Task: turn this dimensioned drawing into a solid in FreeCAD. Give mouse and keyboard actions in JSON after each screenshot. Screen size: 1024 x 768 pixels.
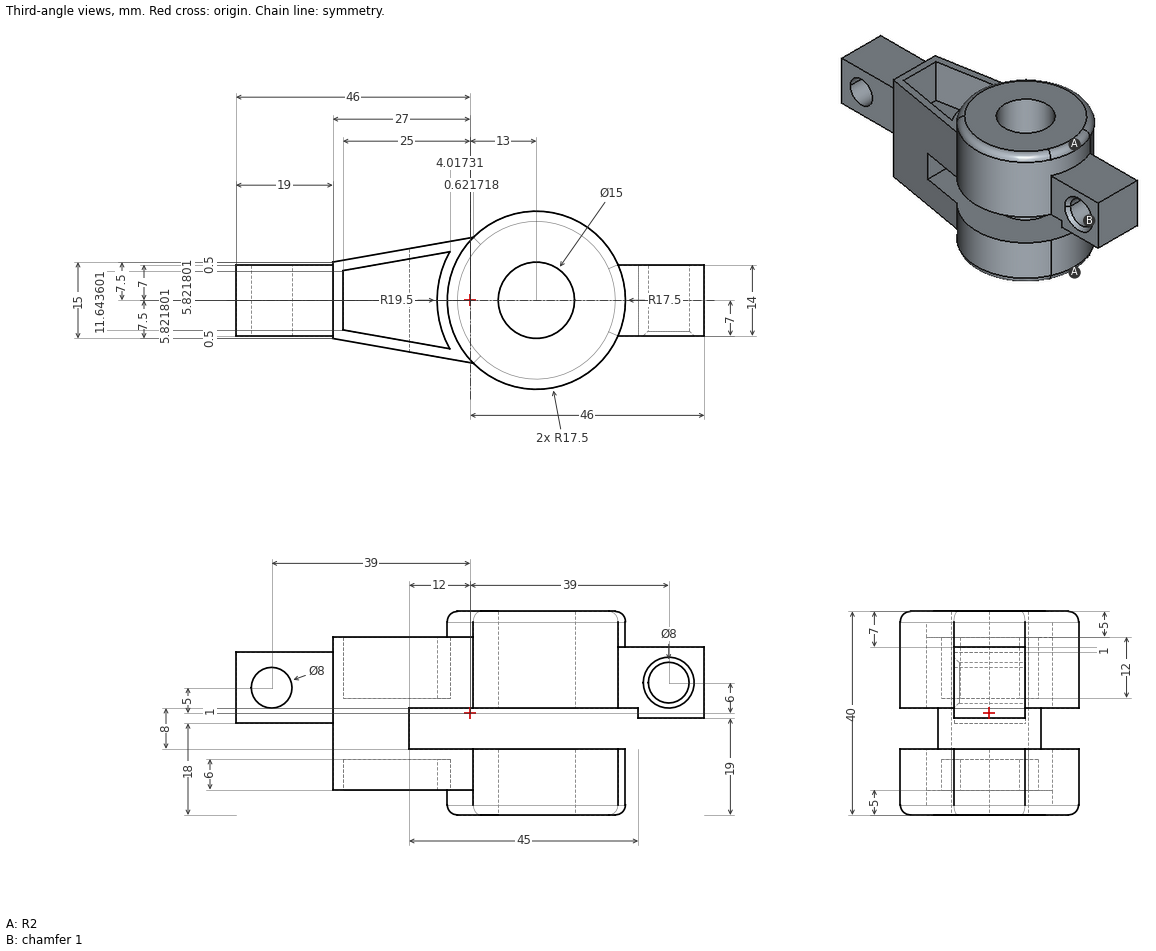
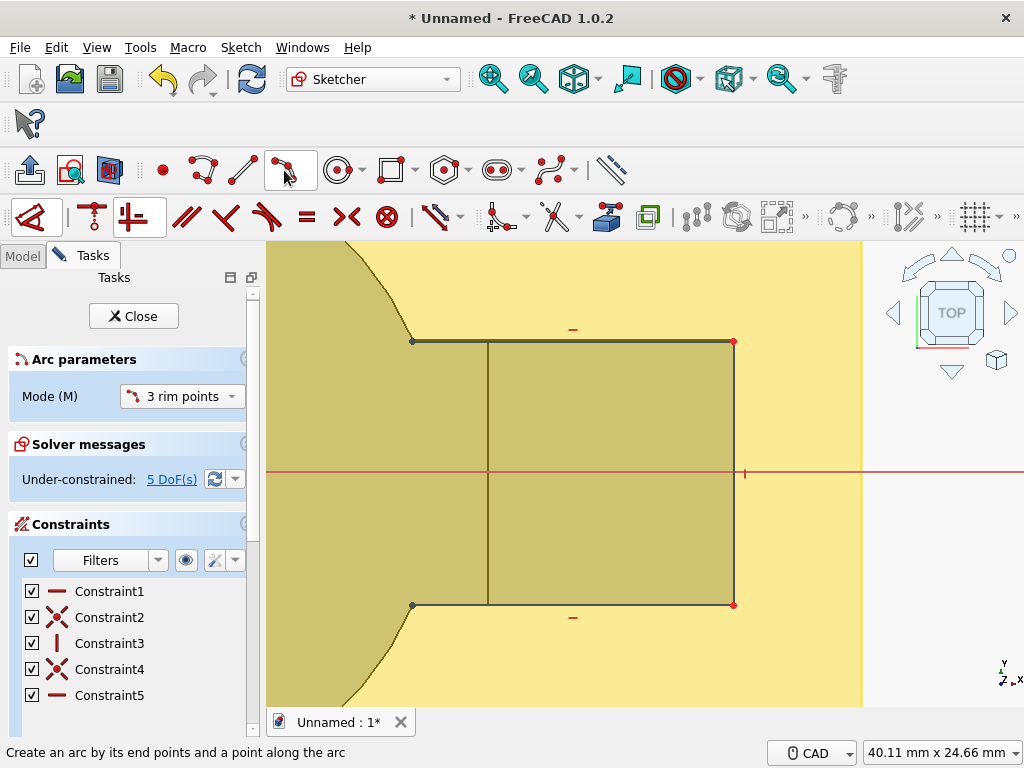
{"action": "left_click", "coordinate": [413, 605]}
{"action": "left_click", "coordinate": [413, 342]}
{"action": "left_click", "coordinate": [440, 500]}
{"action": "key", "text": "Escape"}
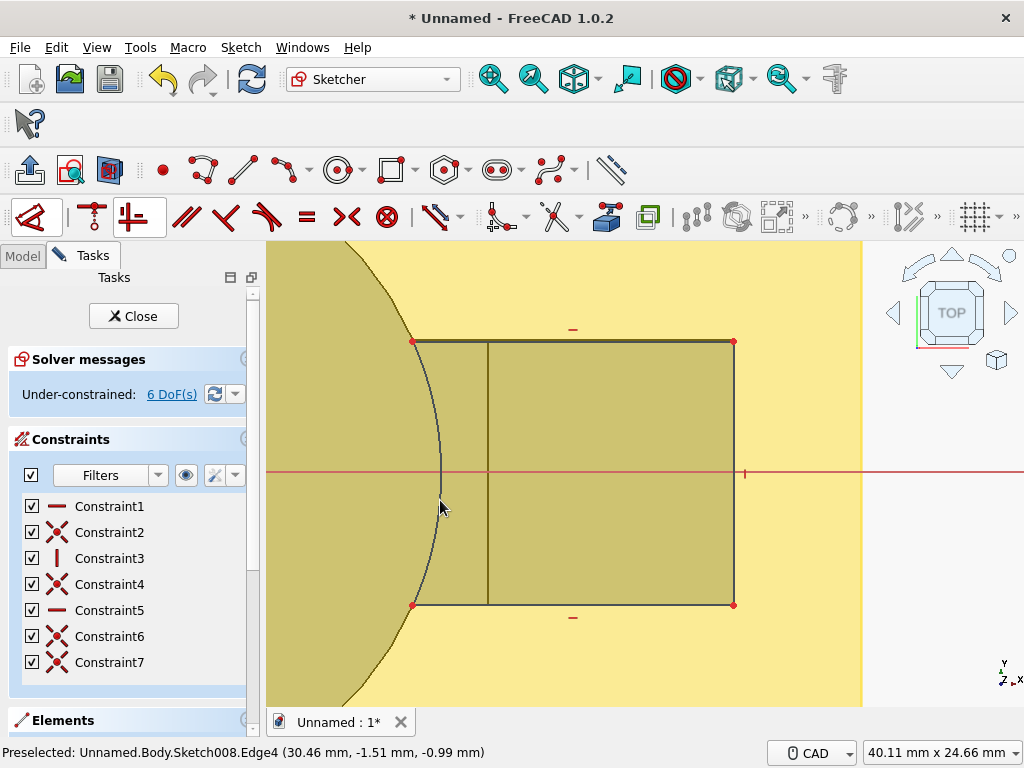
{"action": "scroll", "coordinate": [859, 477], "scroll_direction": "down", "scroll_amount": 2}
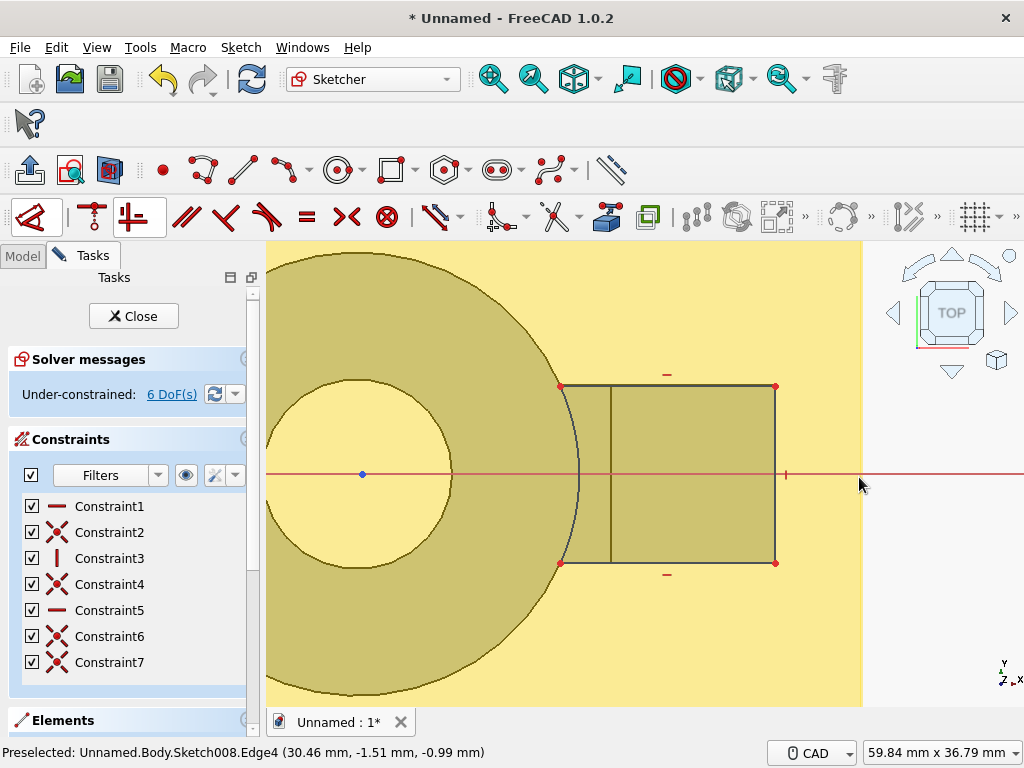
{"action": "left_click", "coordinate": [363, 475]}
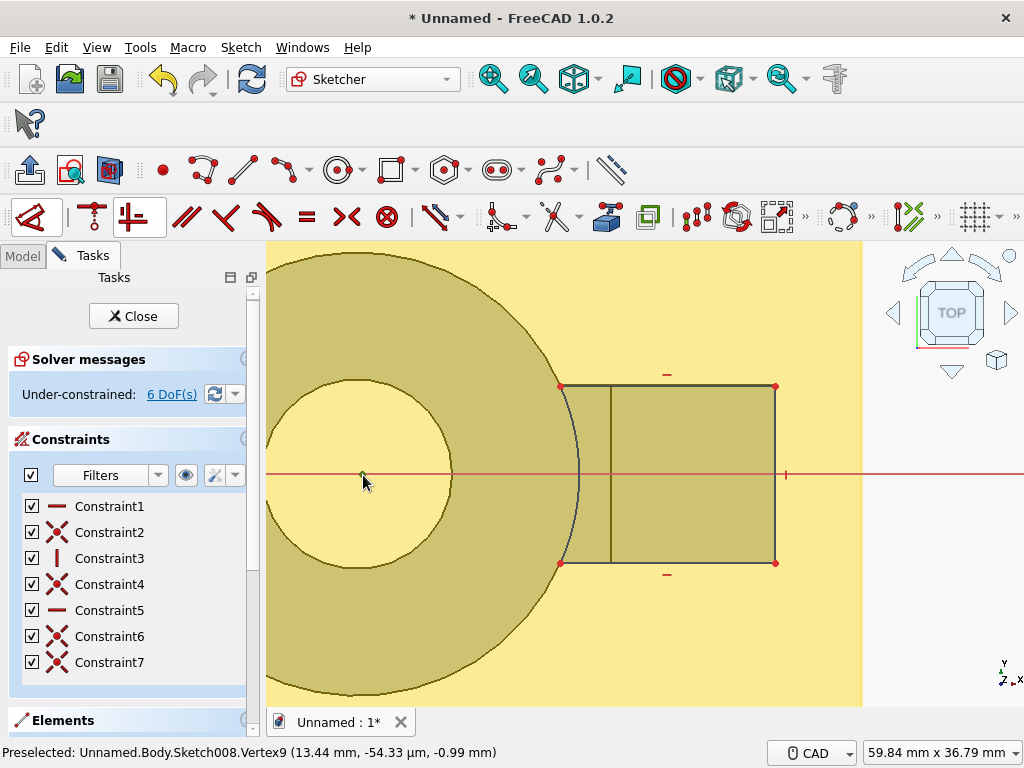
{"action": "left_click", "coordinate": [334, 474]}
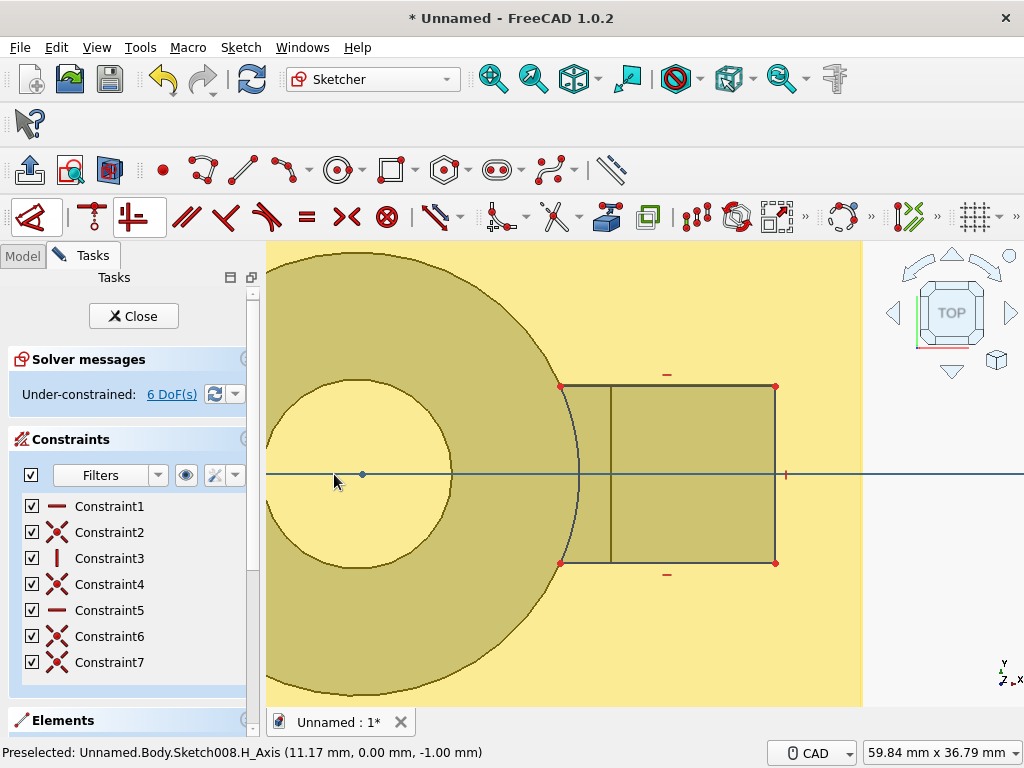
{"action": "left_click", "coordinate": [92, 218]}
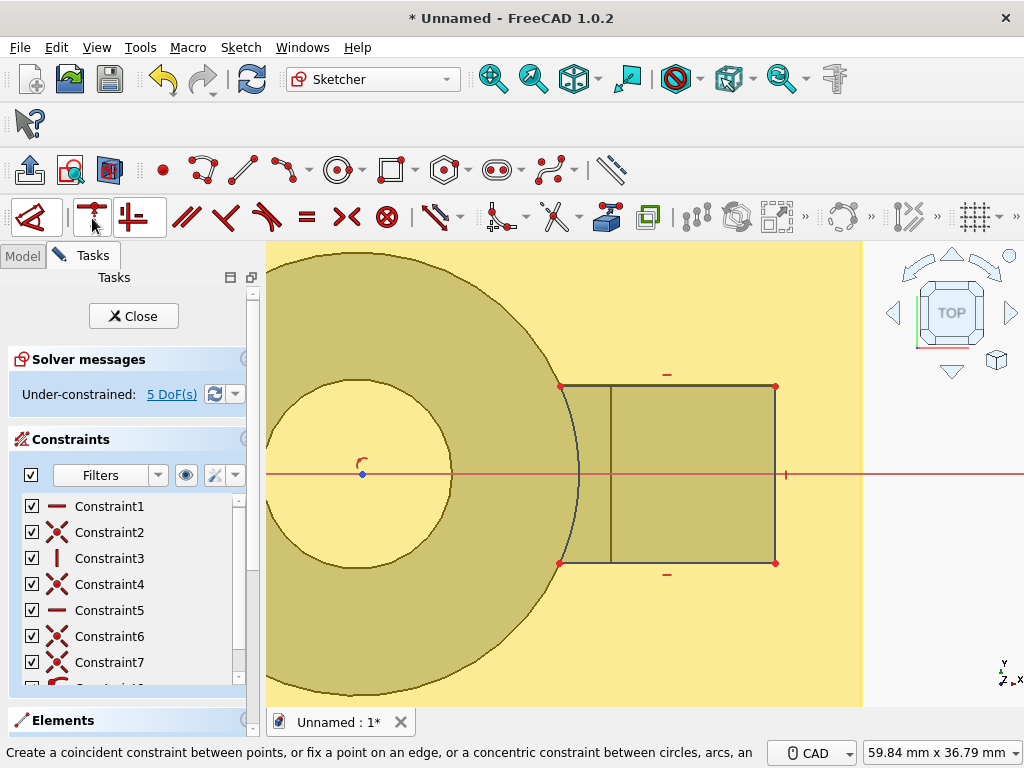
{"action": "left_click", "coordinate": [576, 511]}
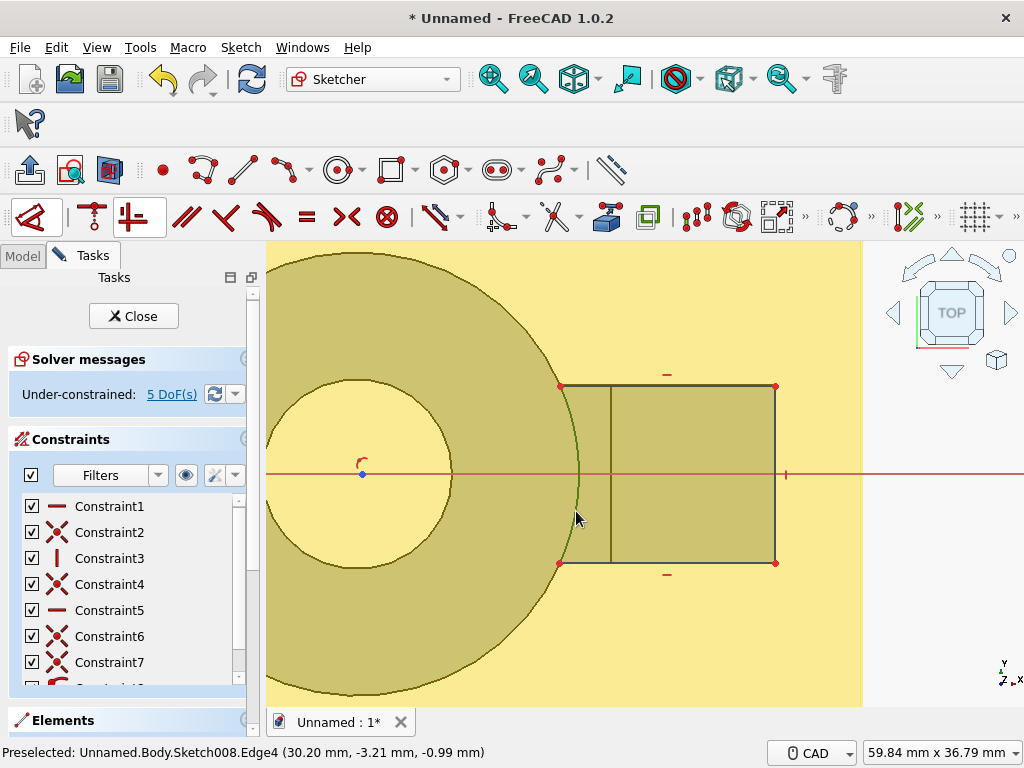
{"action": "key", "text": "k r"}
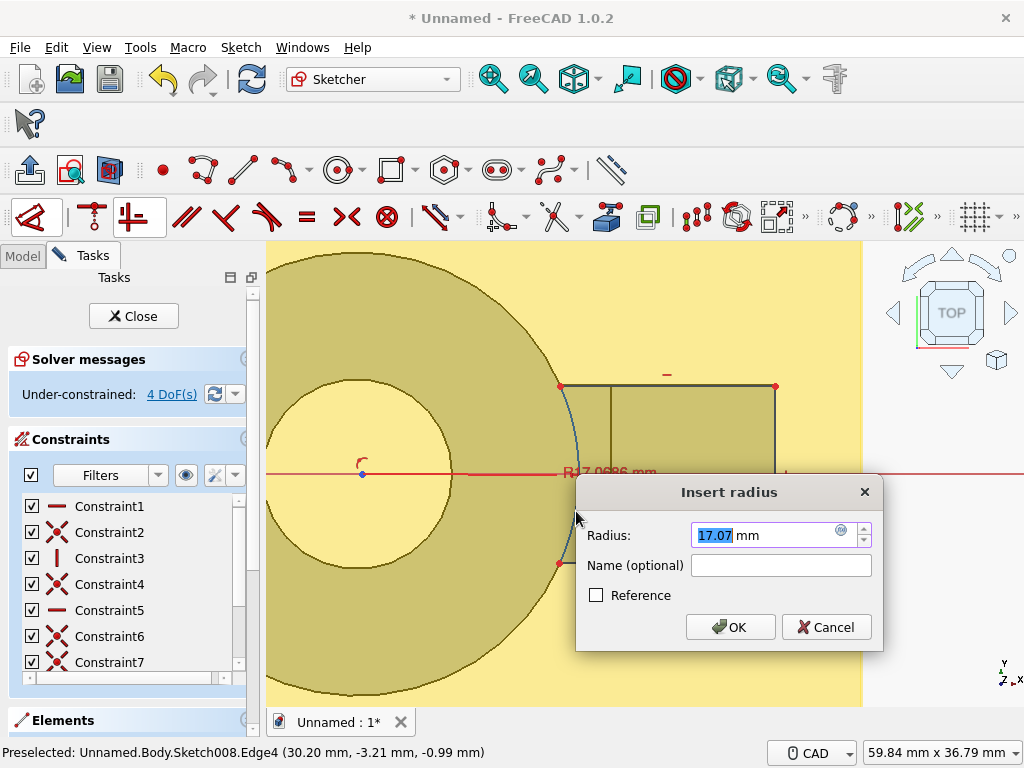
{"action": "type", "text": "17.5"}
{"action": "key", "text": "Return"}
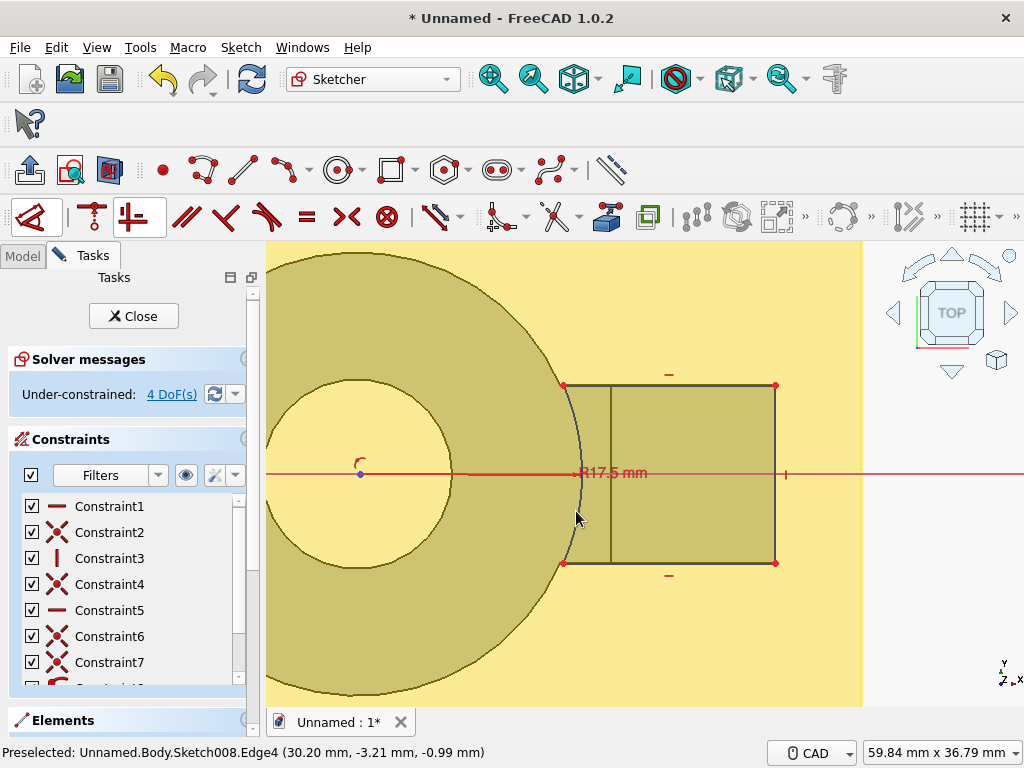
{"action": "left_click", "coordinate": [775, 439]}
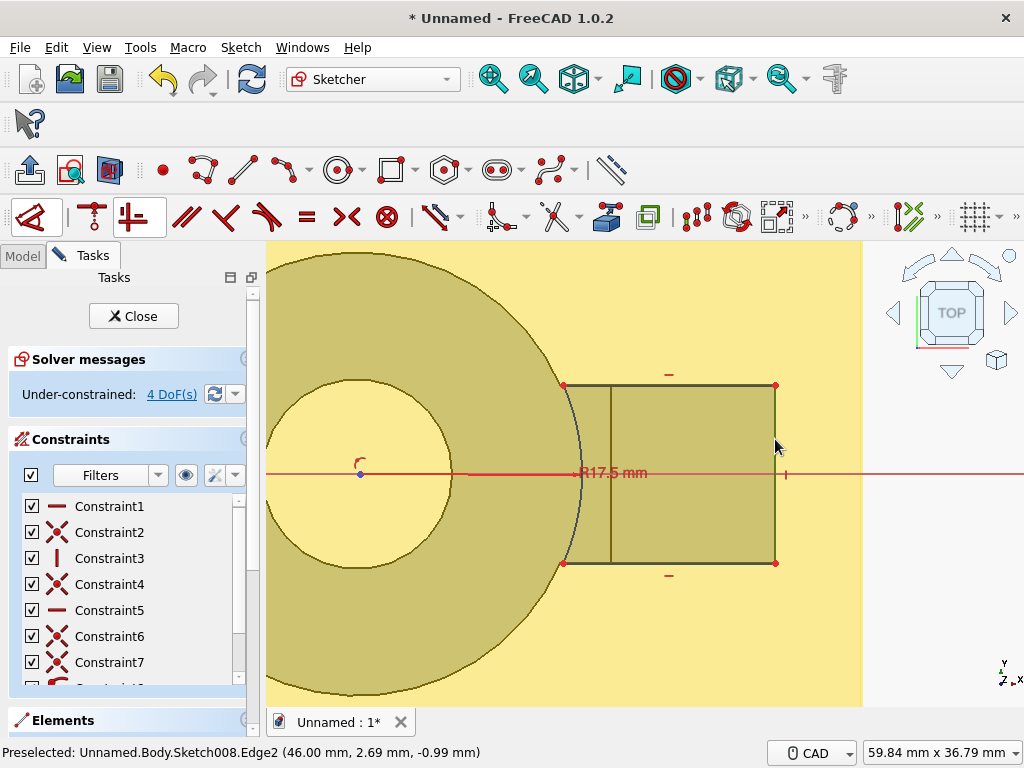
{"action": "left_click", "coordinate": [56, 218]}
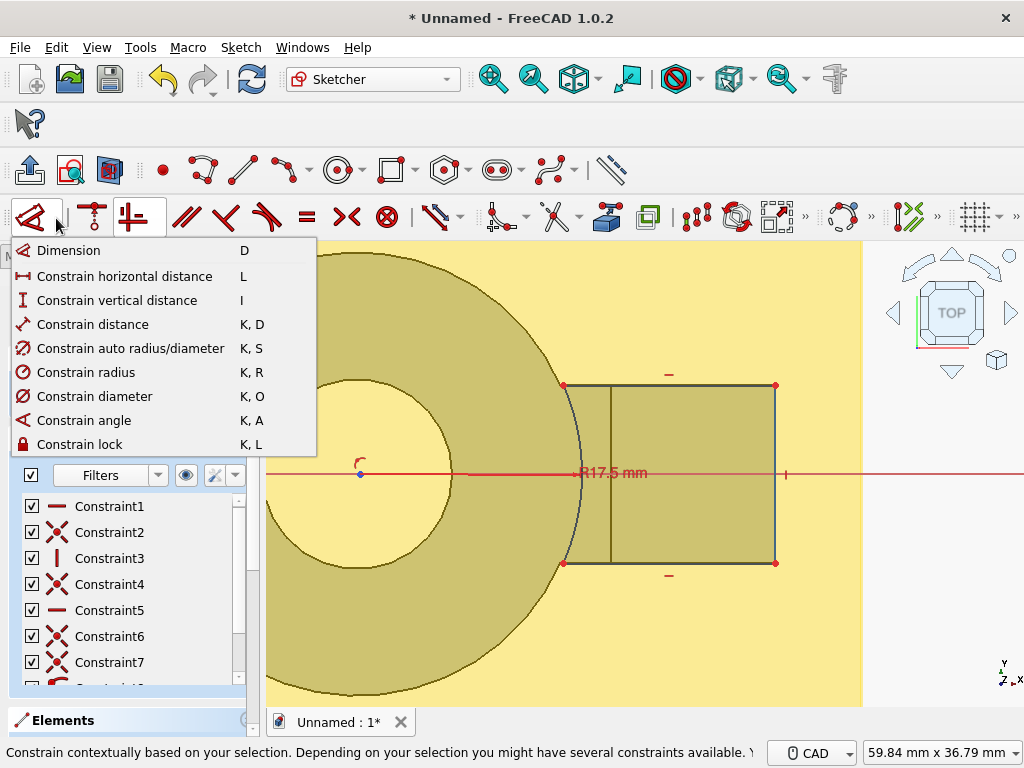
{"action": "left_click", "coordinate": [164, 300]}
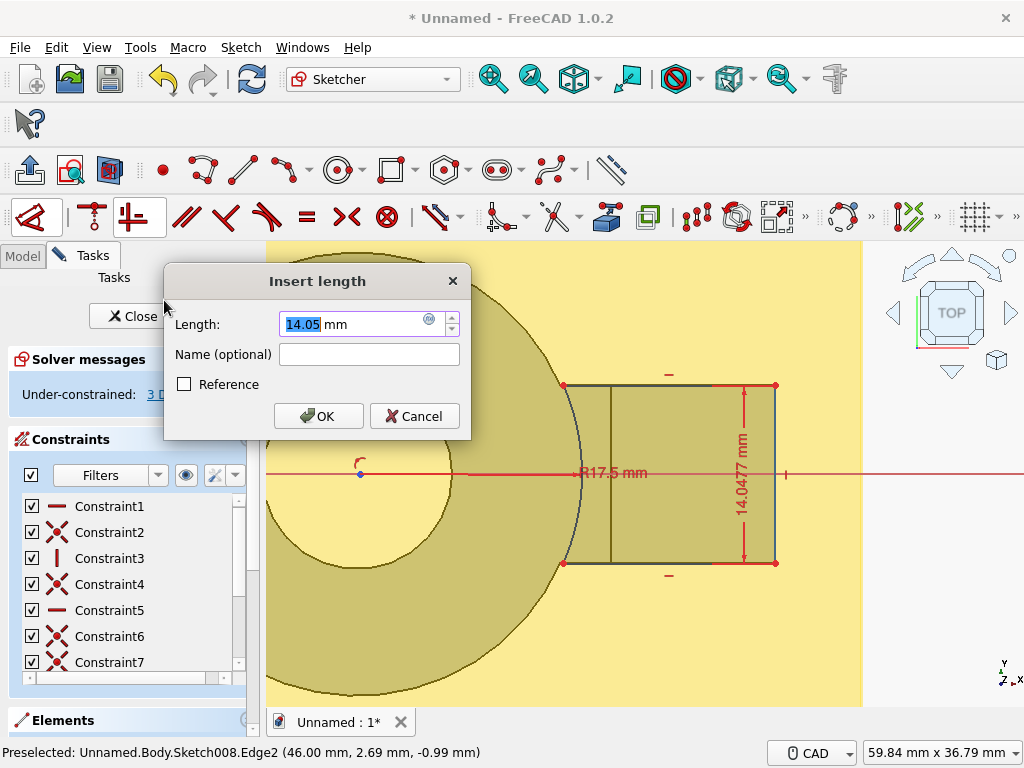
{"action": "type", "text": "14"}
{"action": "key", "text": "Return"}